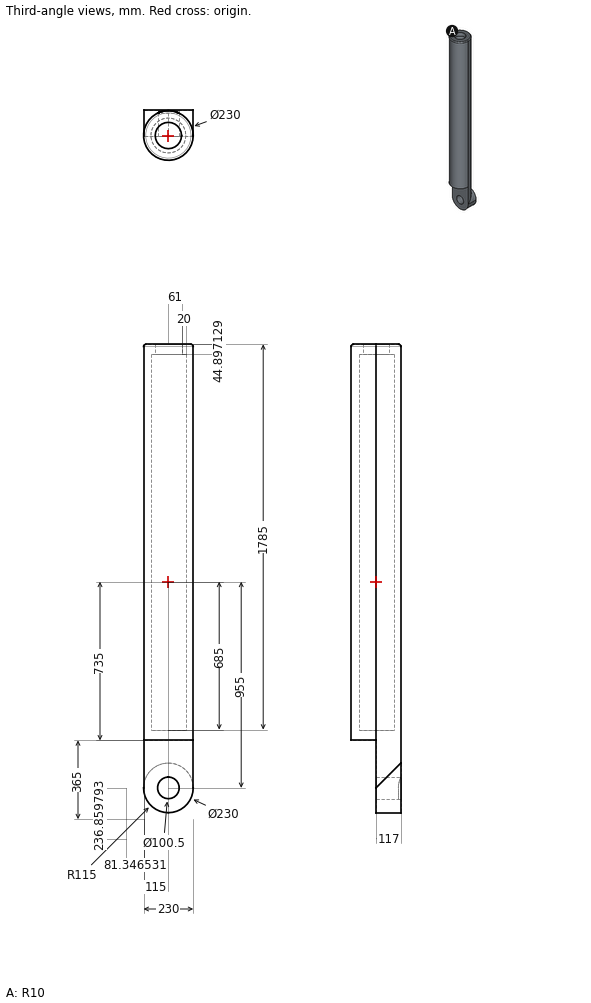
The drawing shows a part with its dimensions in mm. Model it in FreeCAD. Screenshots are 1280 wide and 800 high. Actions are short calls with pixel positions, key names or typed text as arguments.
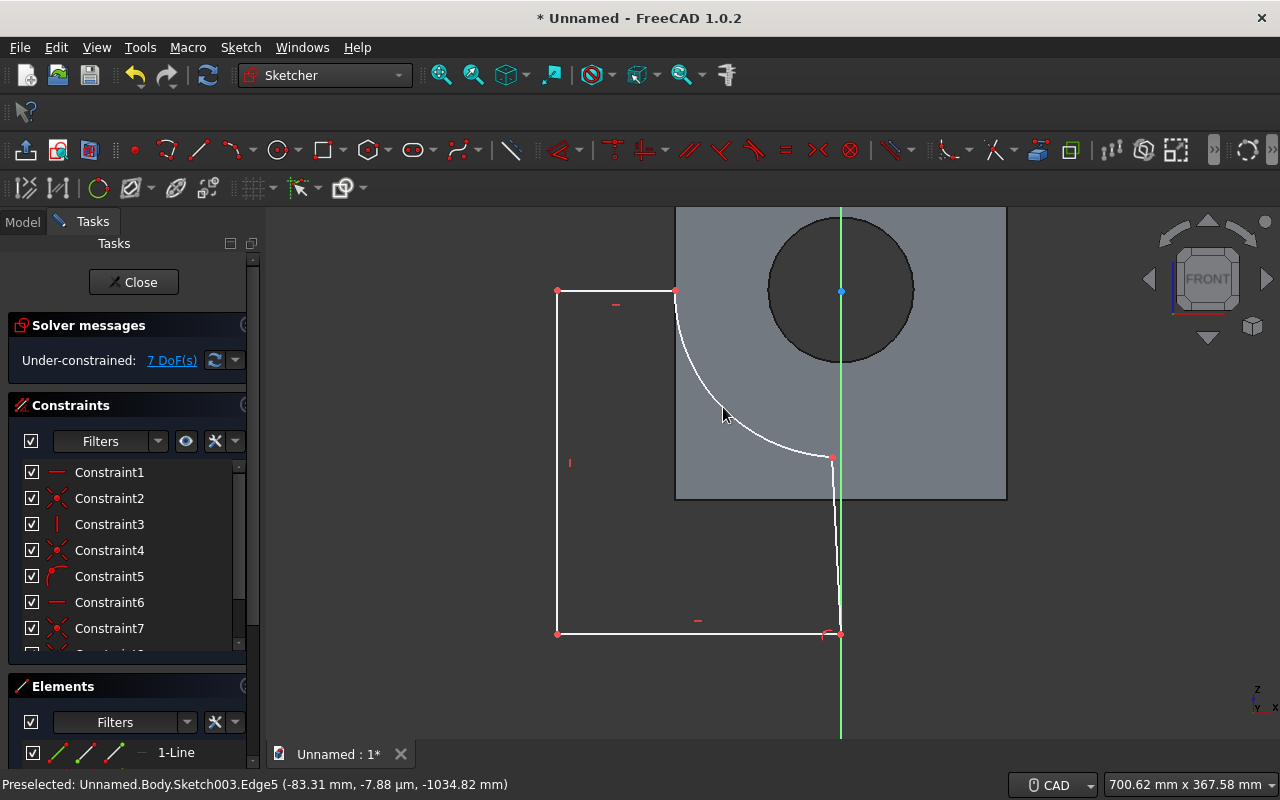
click(838, 581)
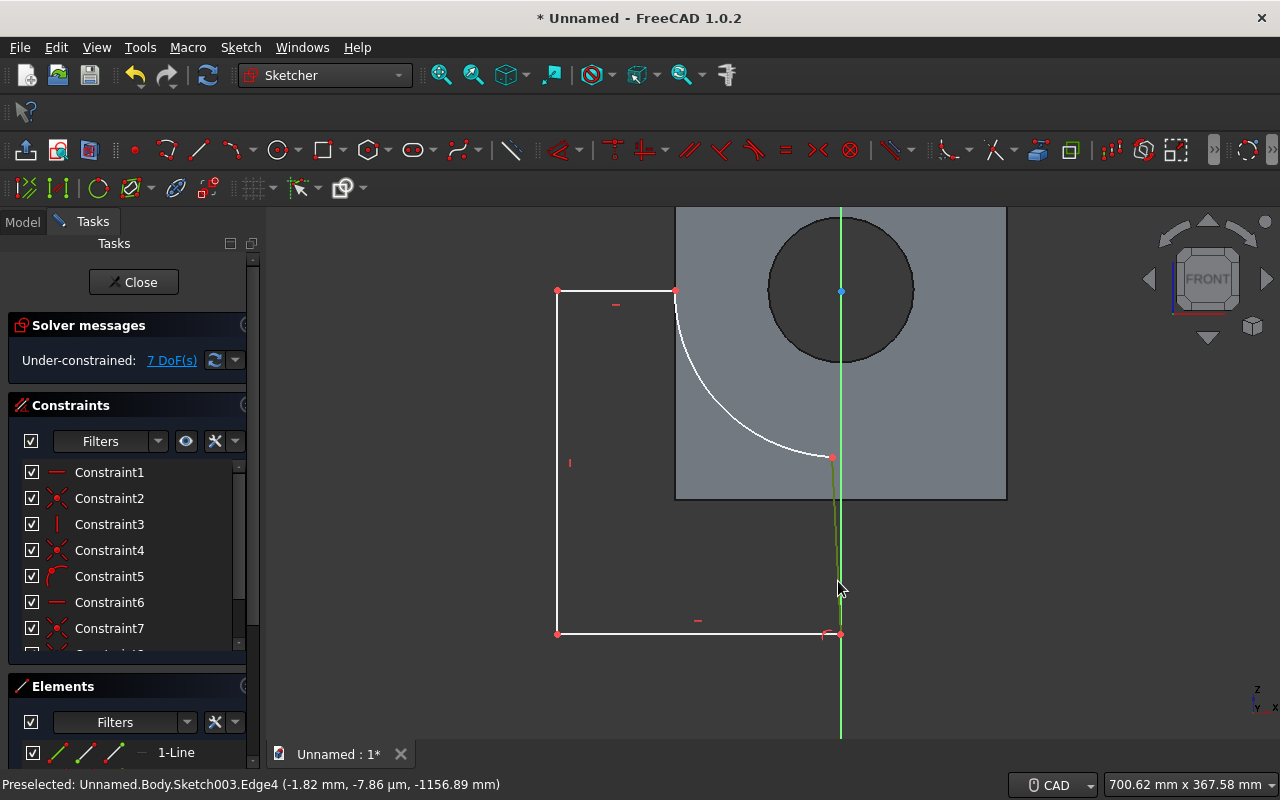
key(v)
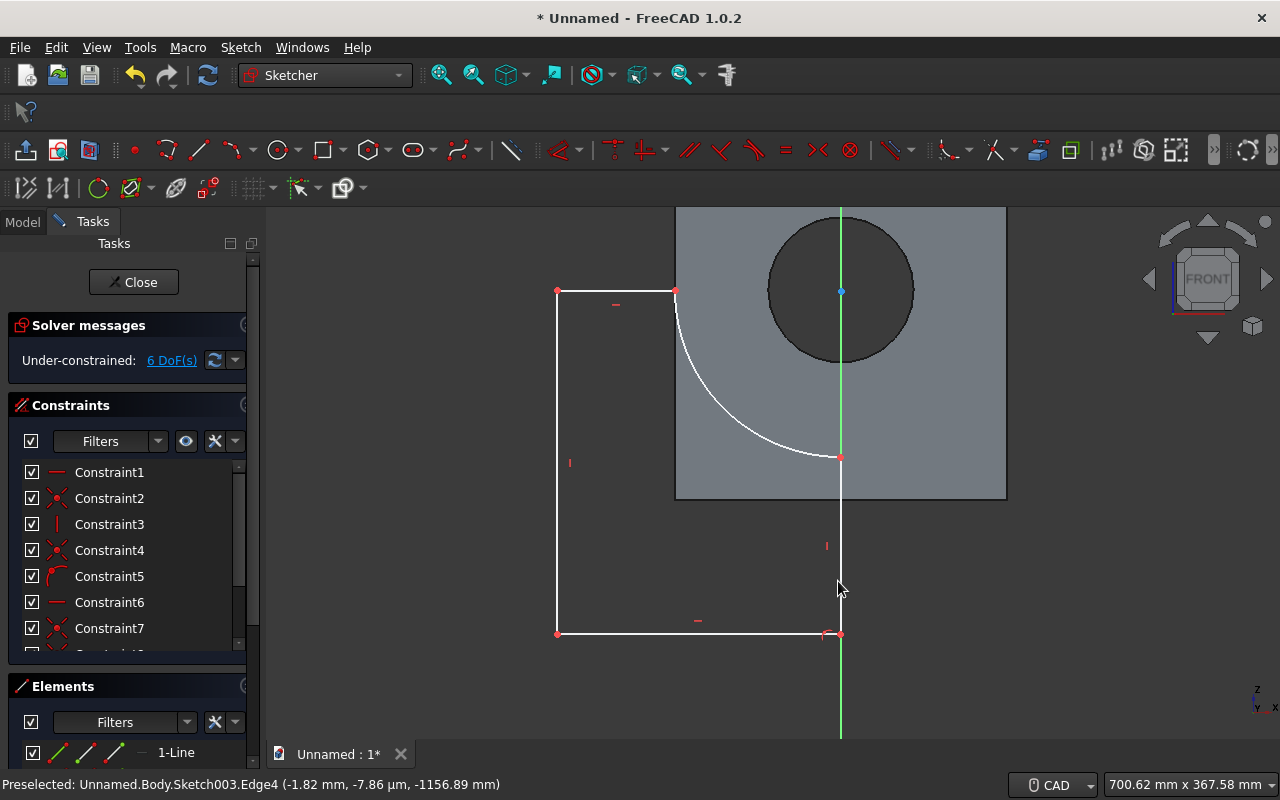
click(841, 291)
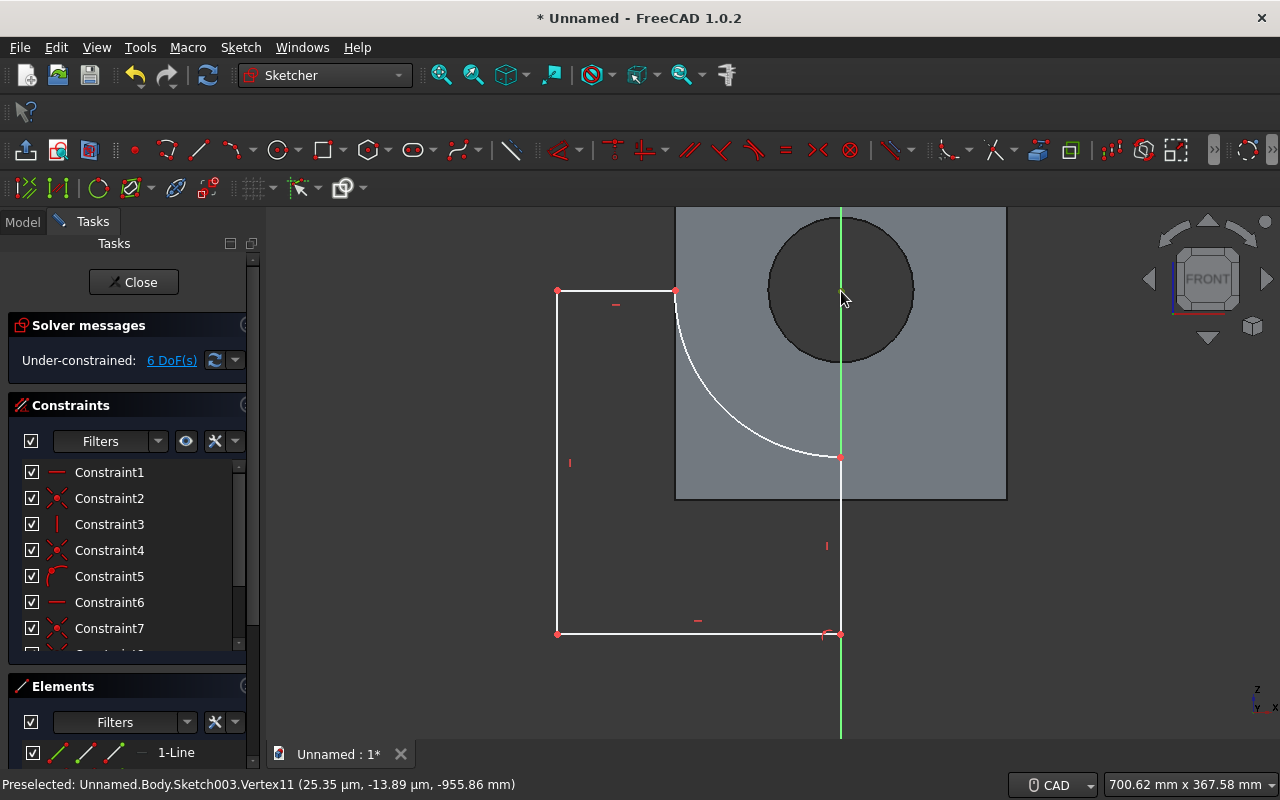
click(841, 677)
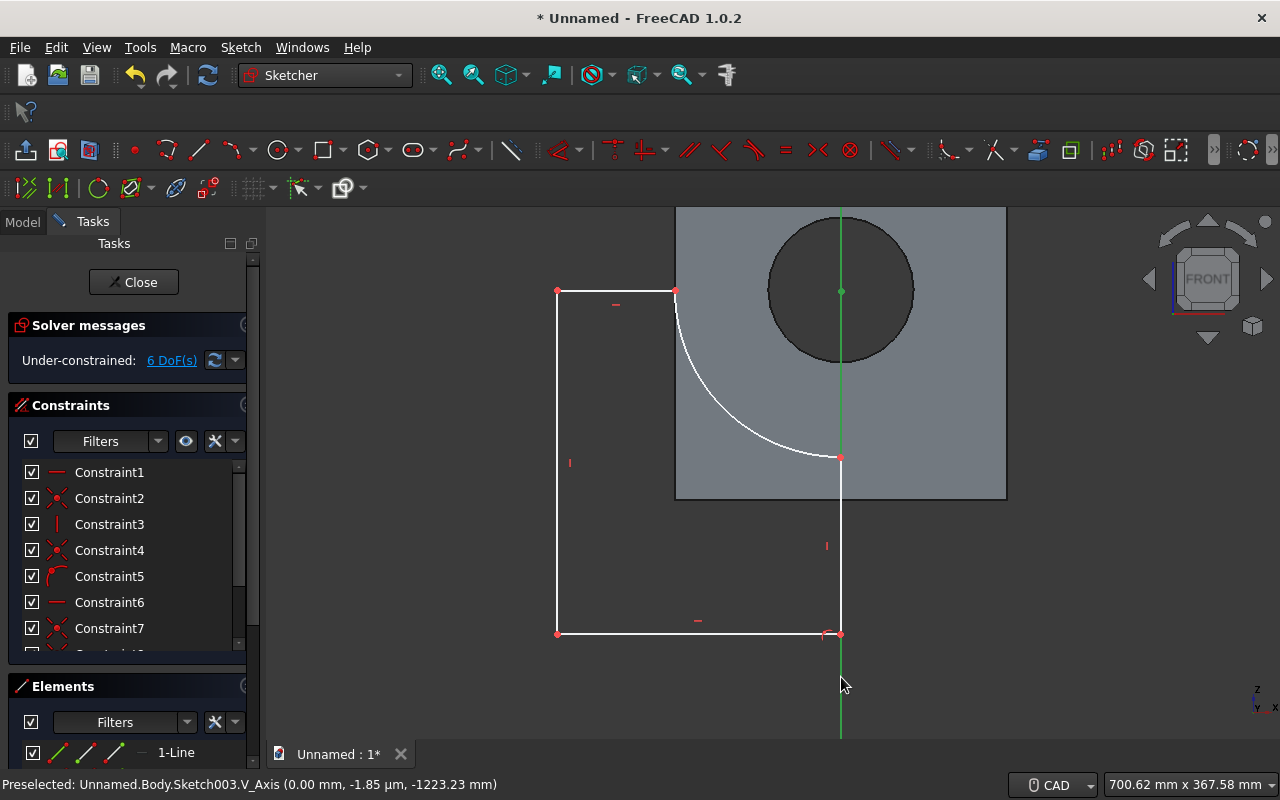
click(614, 150)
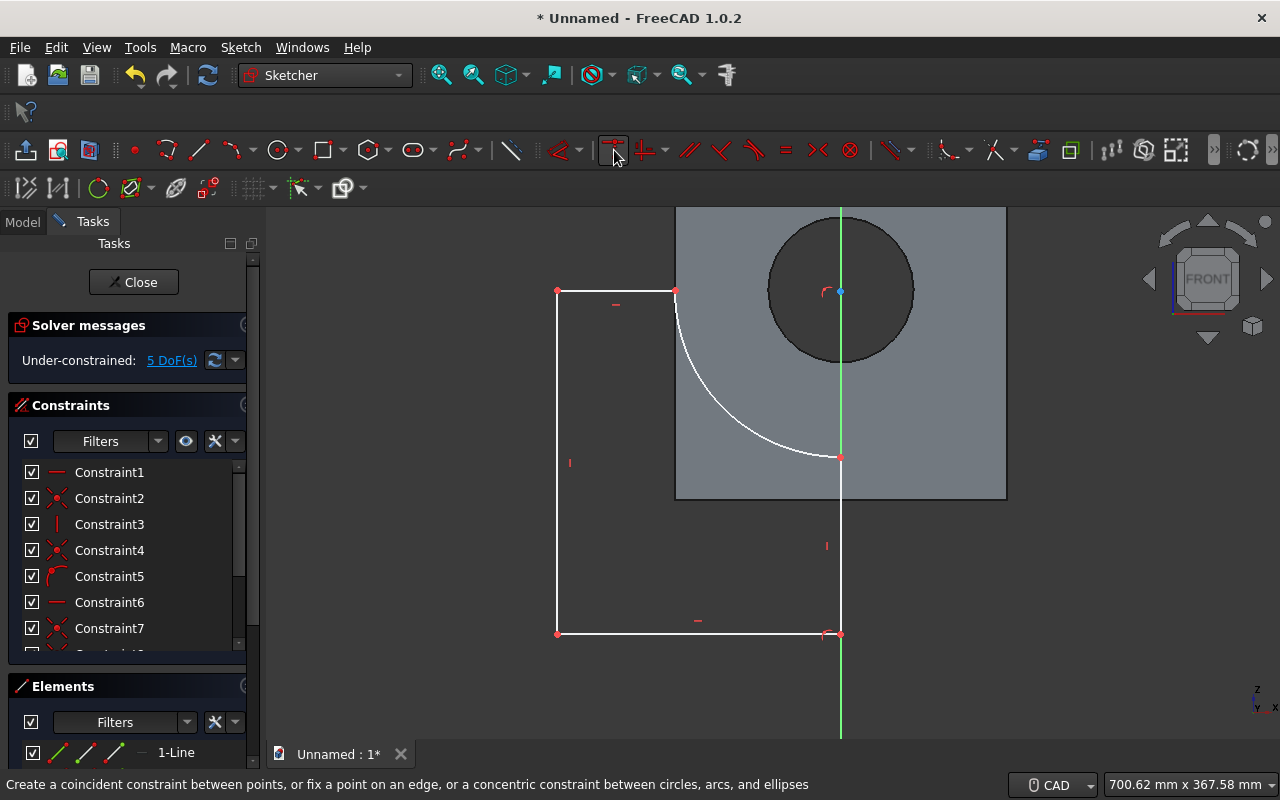
click(558, 150)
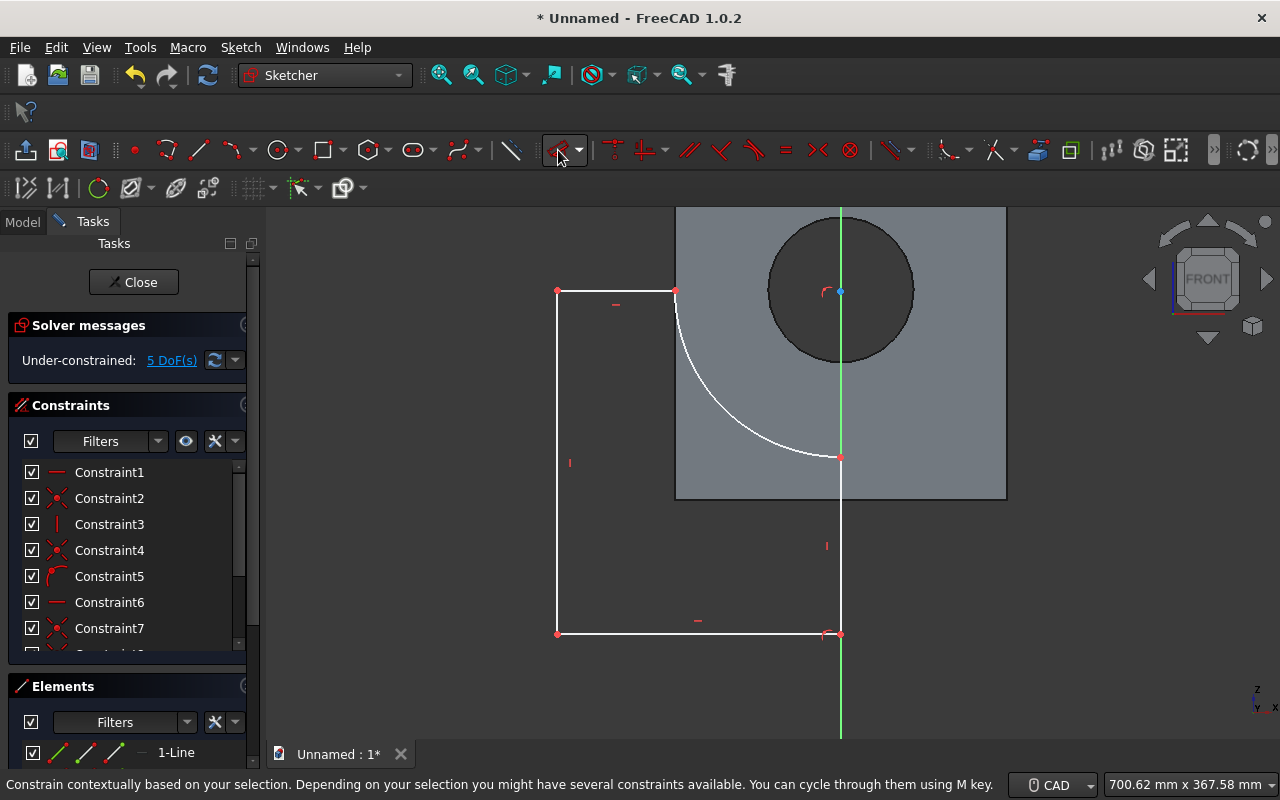
click(693, 366)
click(664, 380)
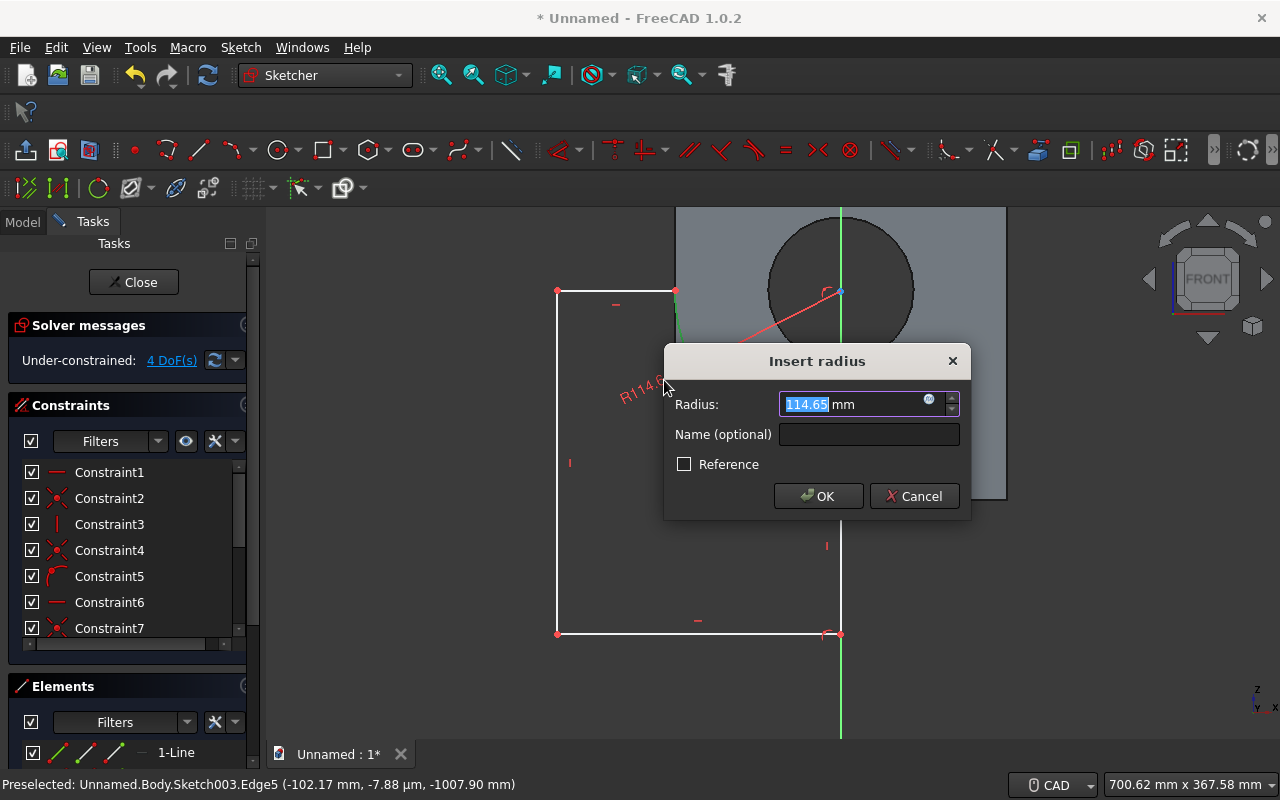
text(115)
key(Return)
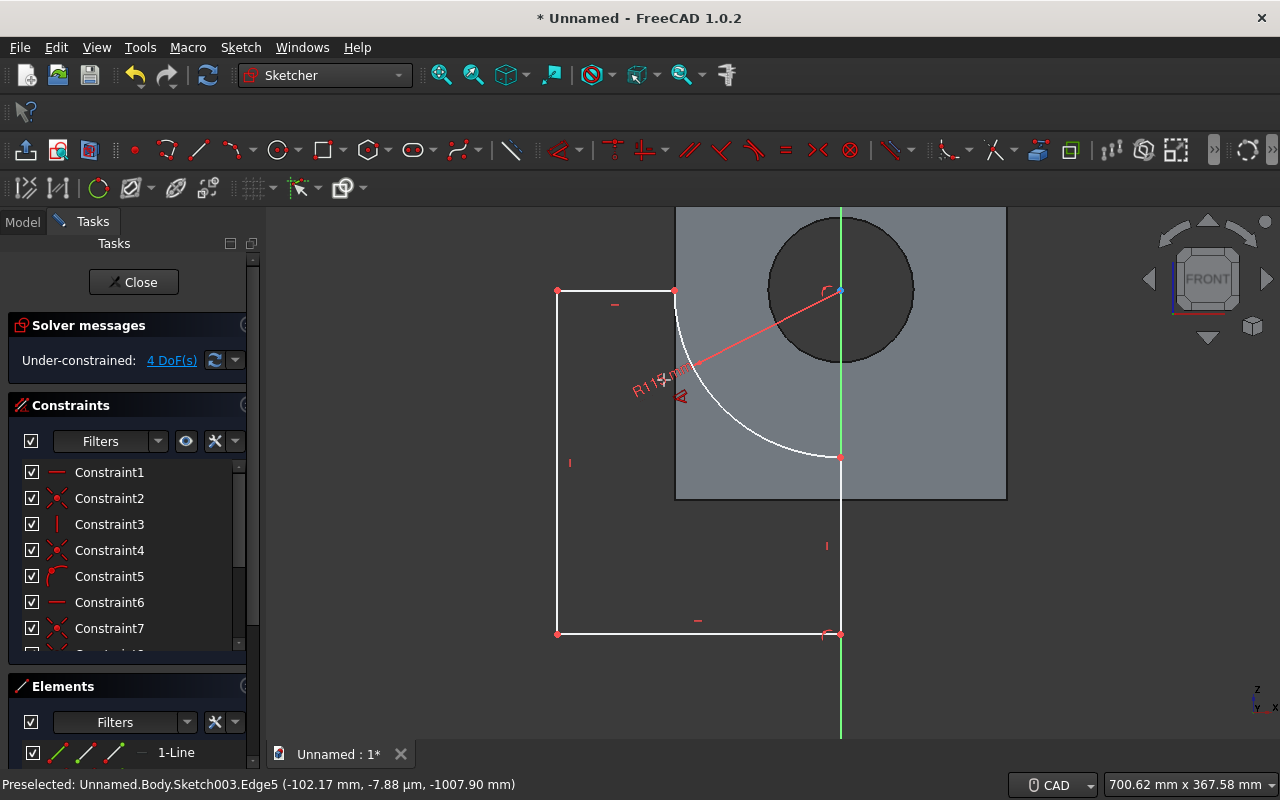
click(675, 291)
click(875, 263)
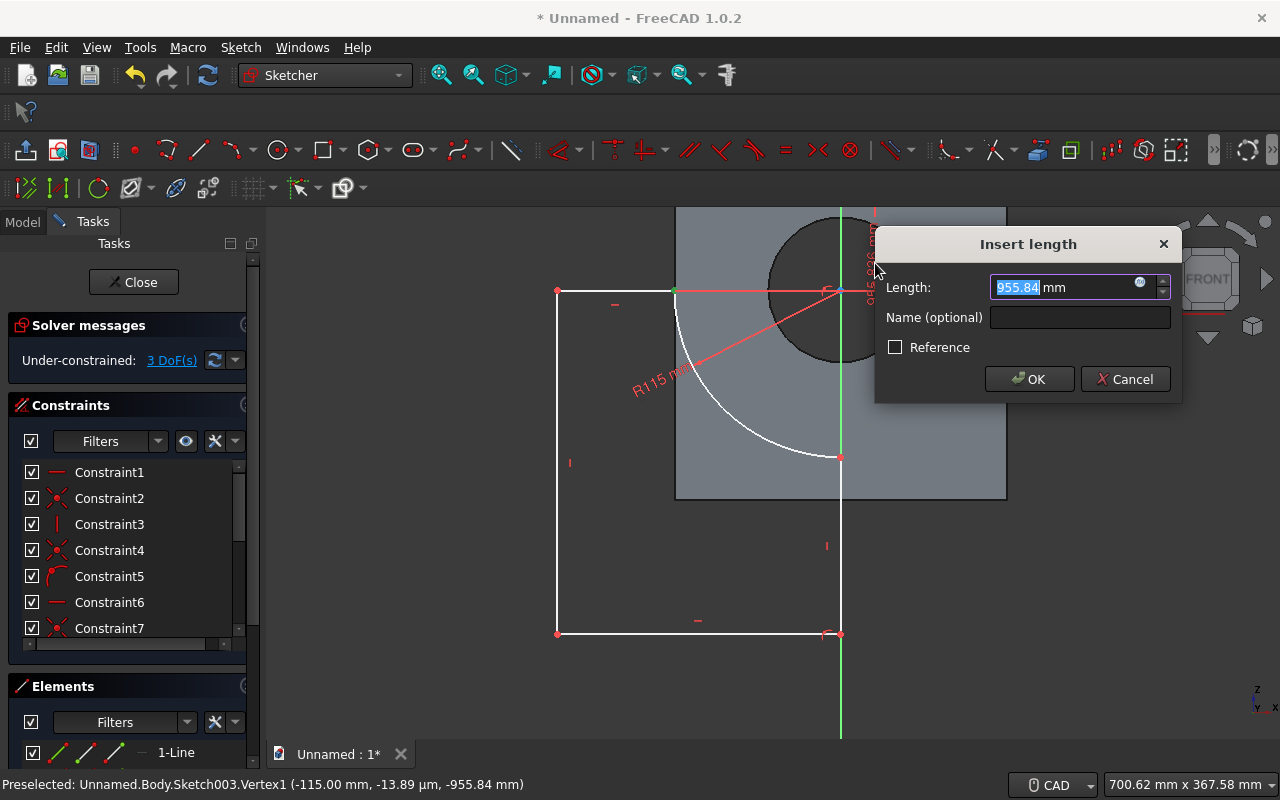
text(955)
key(Return)